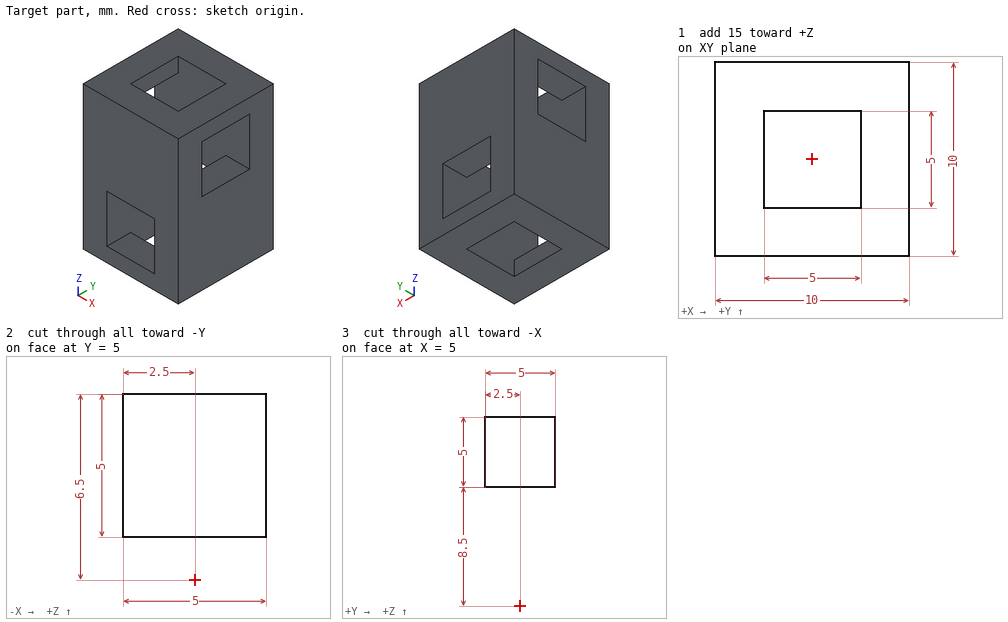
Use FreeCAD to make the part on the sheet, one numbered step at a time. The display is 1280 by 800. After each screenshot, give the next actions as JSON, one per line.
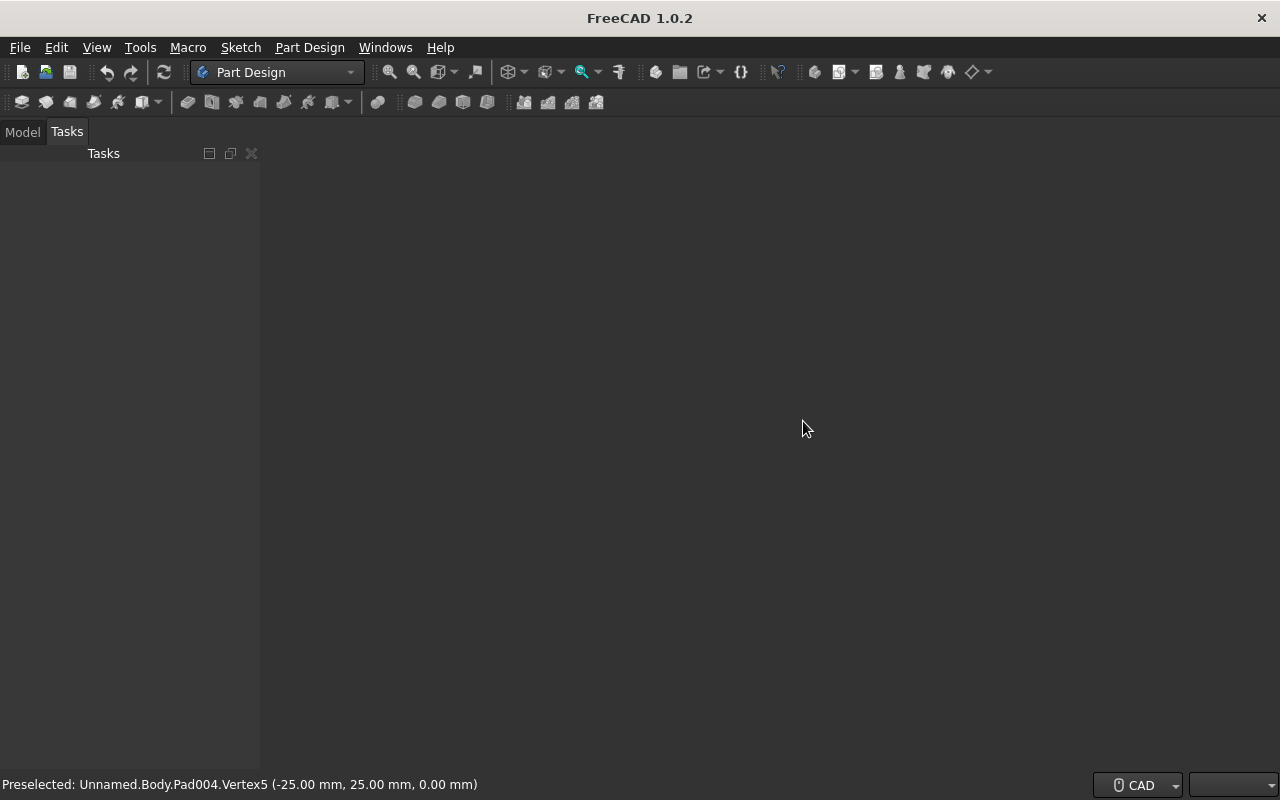
{"action": "left_click", "coordinate": [22, 72]}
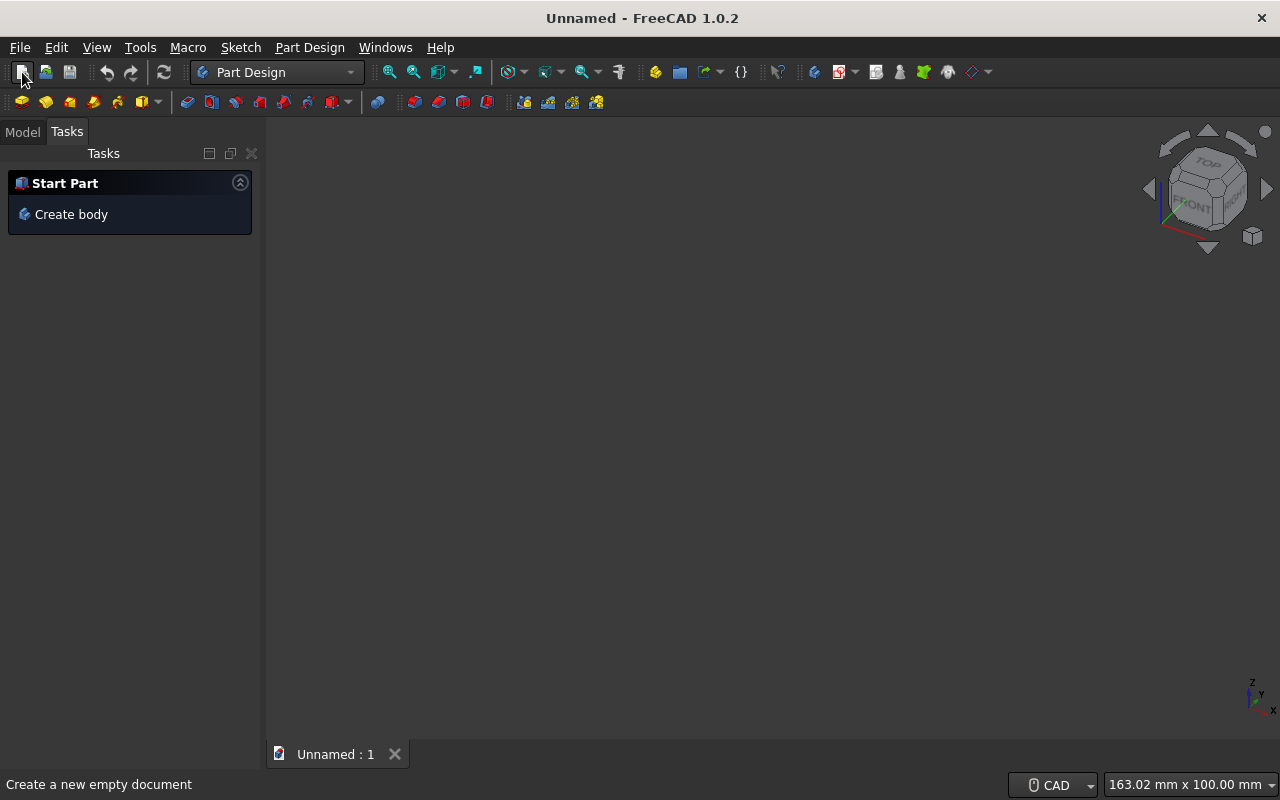
{"action": "left_click", "coordinate": [840, 72]}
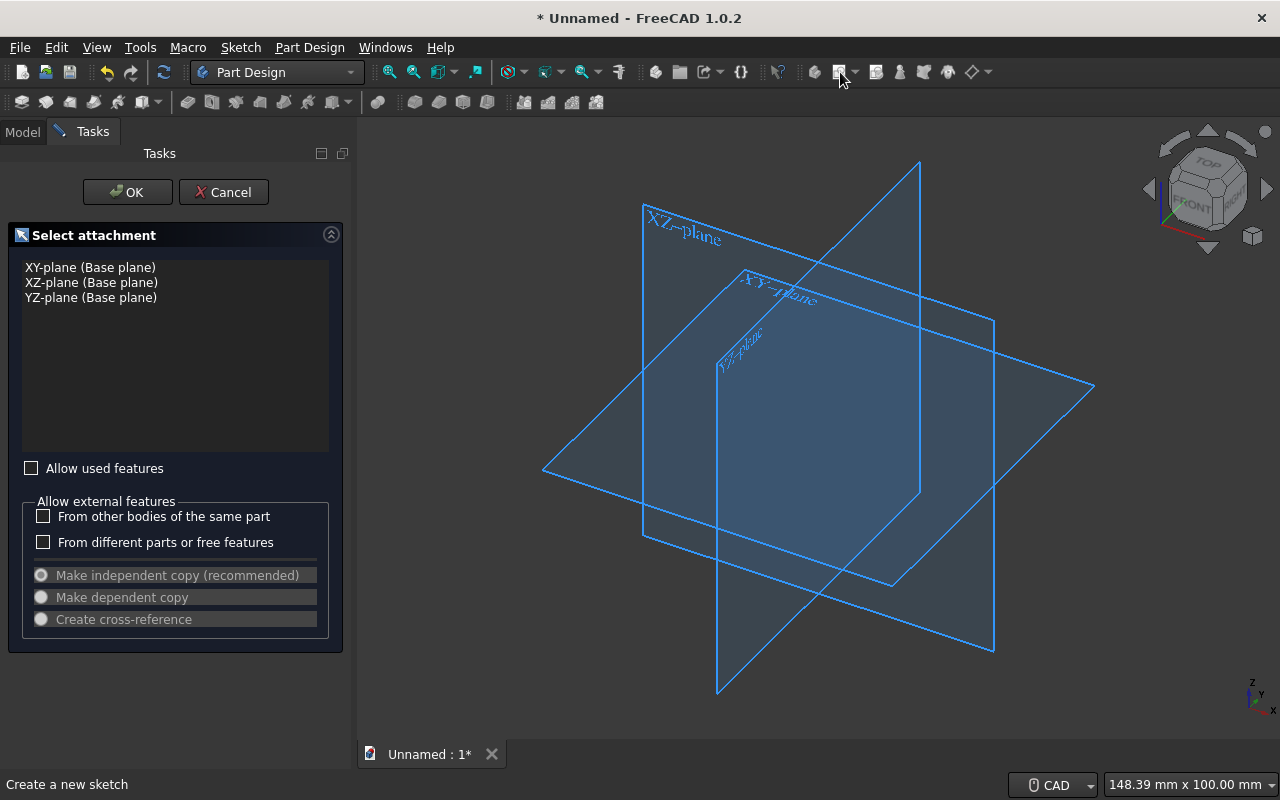
{"action": "left_click", "coordinate": [82, 268]}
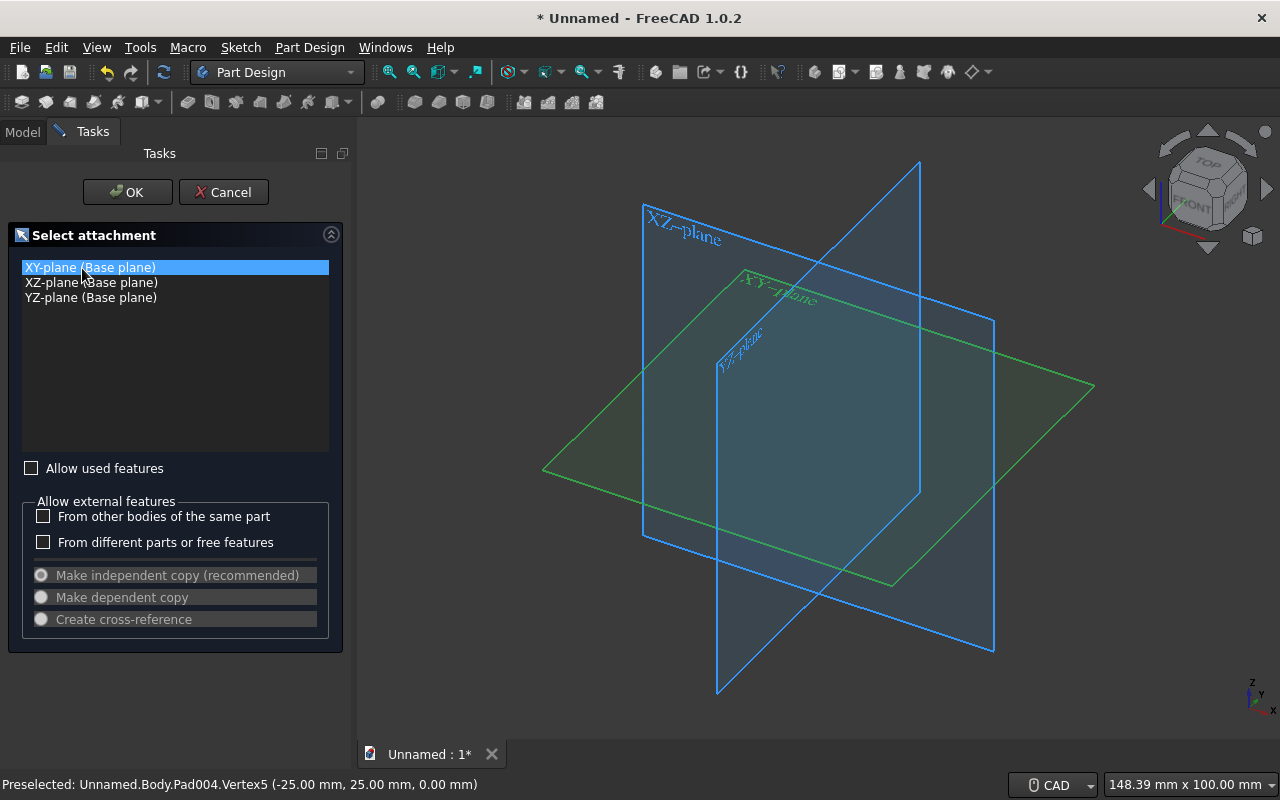
{"action": "left_click", "coordinate": [128, 192]}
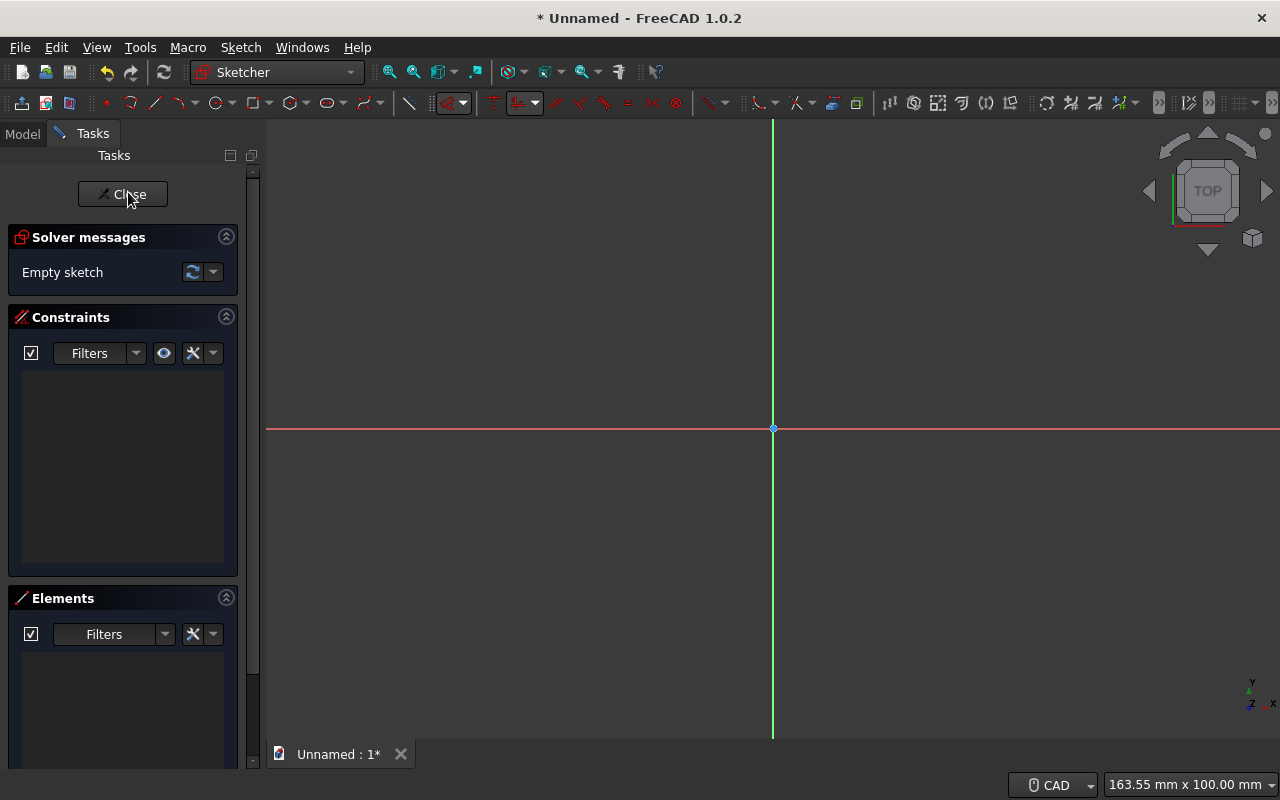
{"action": "scroll", "coordinate": [787, 429], "scroll_direction": "up", "scroll_amount": 9}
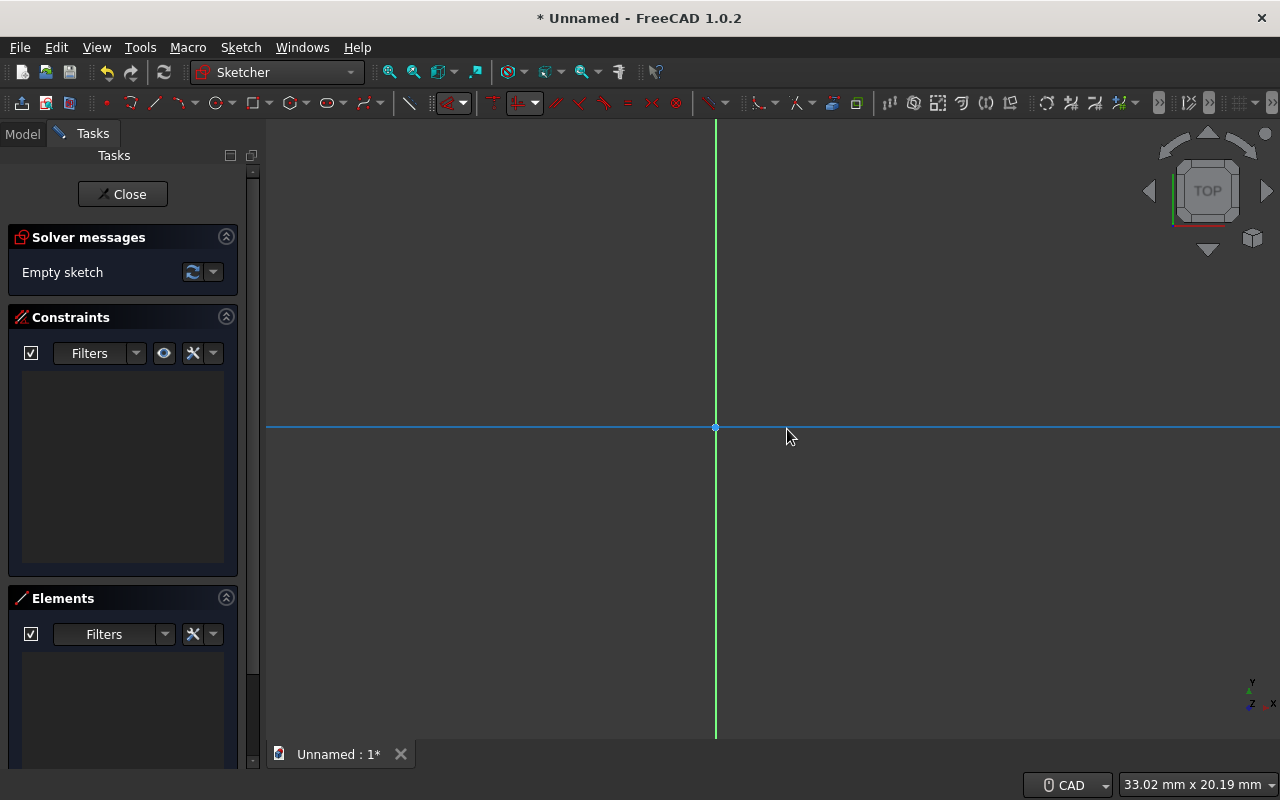
{"action": "left_click", "coordinate": [272, 104]}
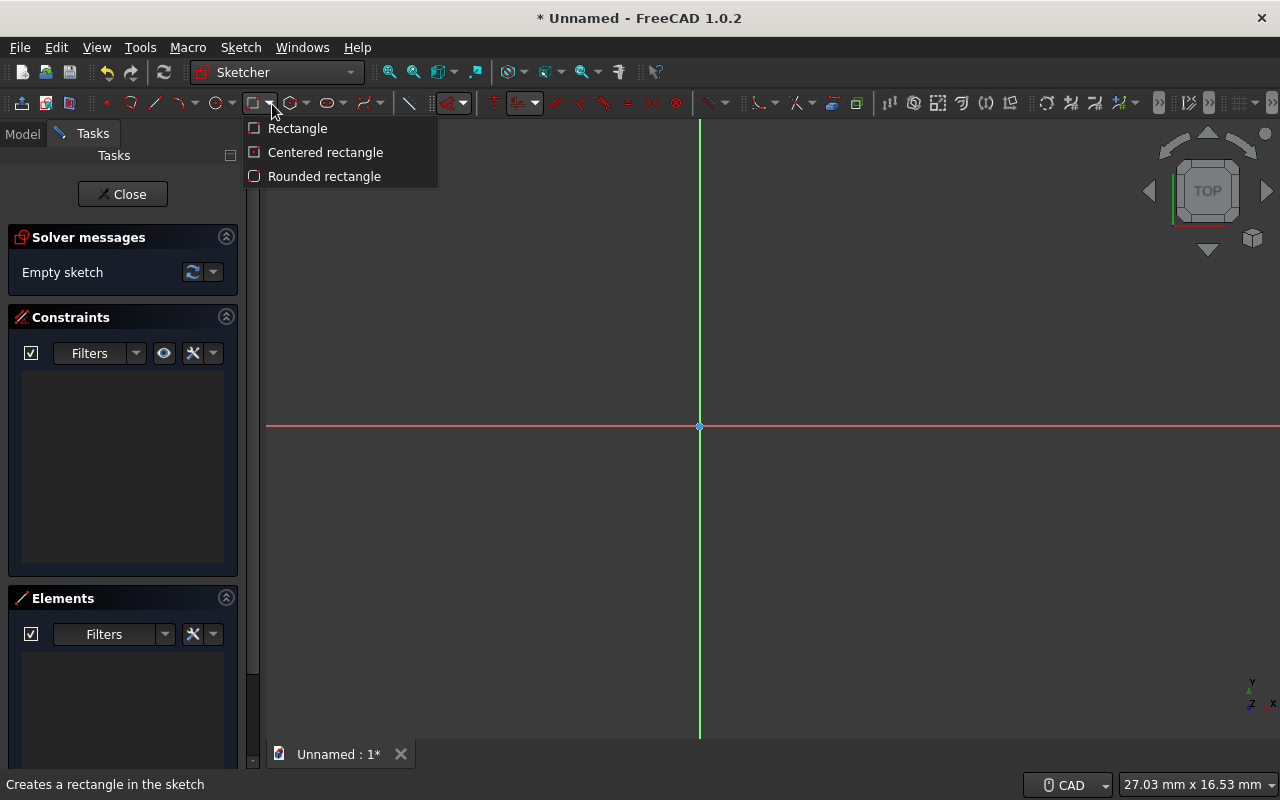
{"action": "left_click", "coordinate": [340, 152]}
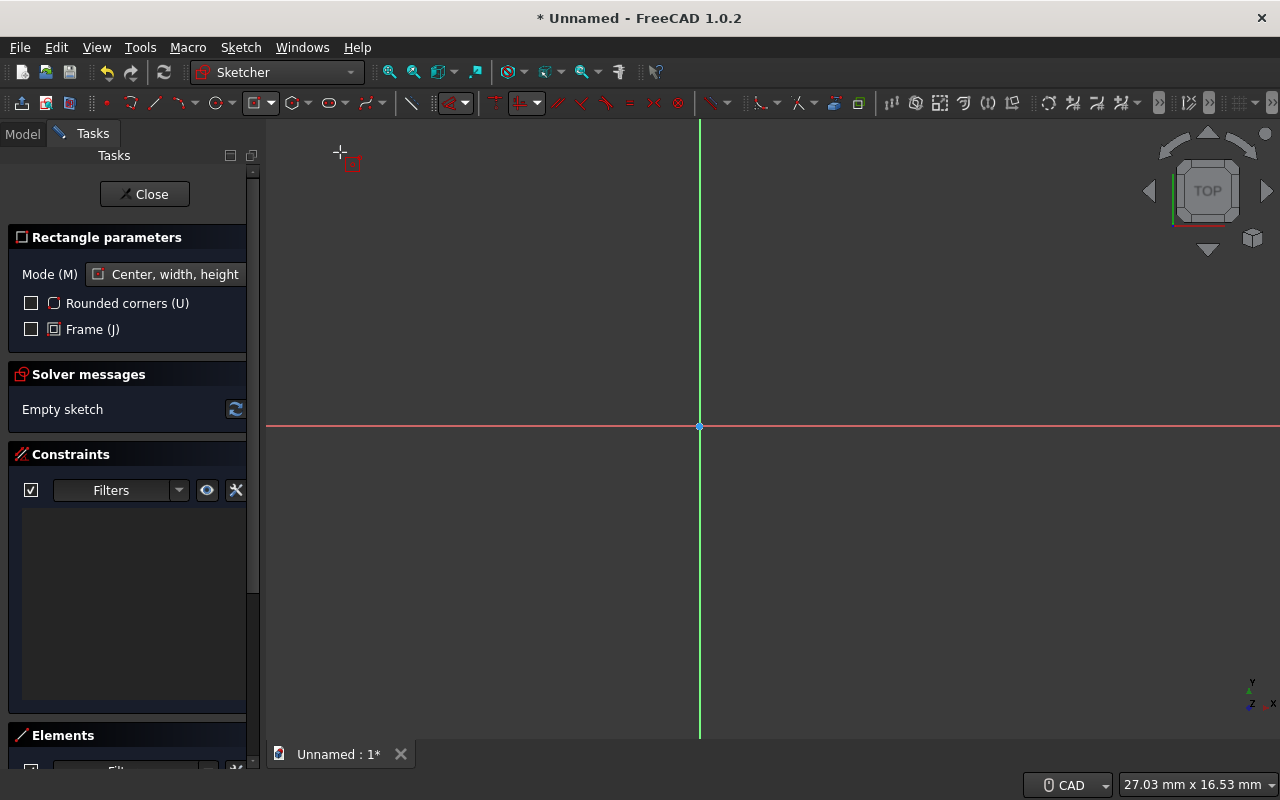
{"action": "left_click", "coordinate": [700, 426]}
{"action": "left_click", "coordinate": [887, 239]}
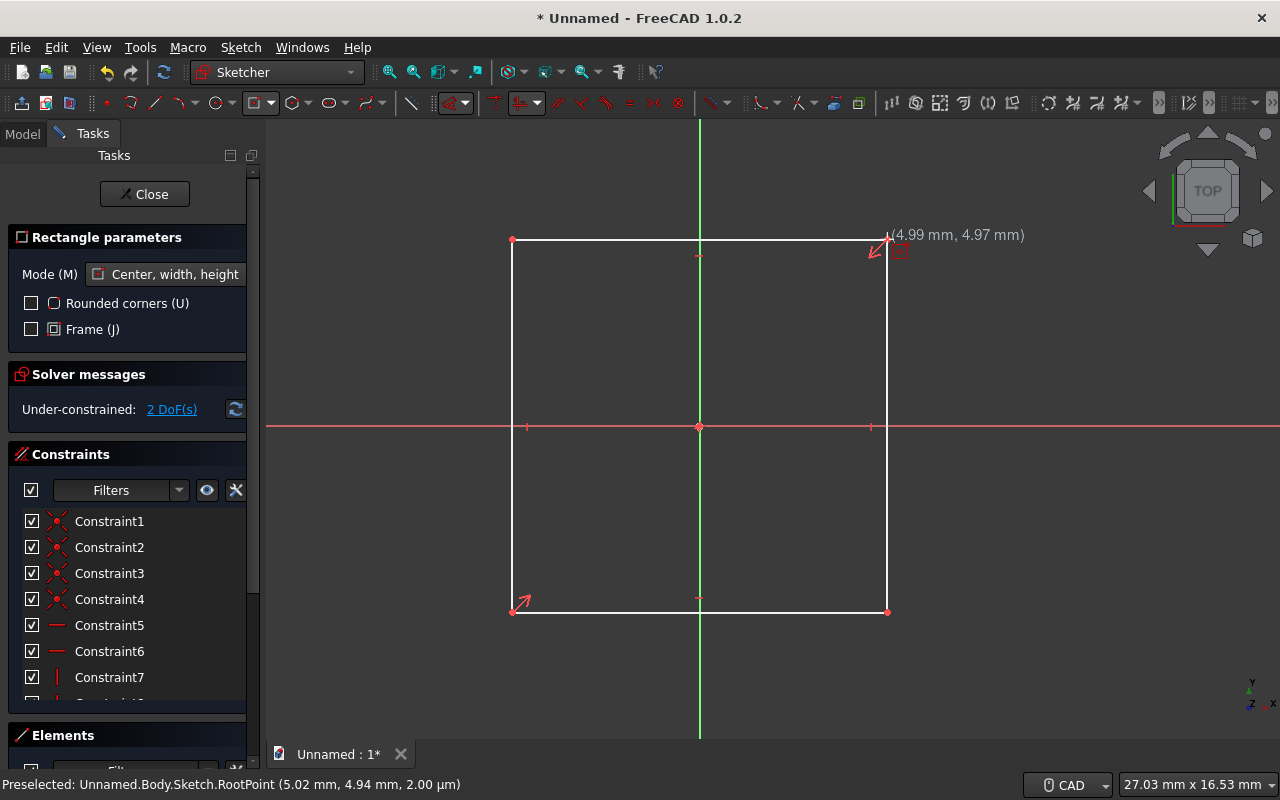
{"action": "left_click", "coordinate": [700, 426]}
{"action": "left_click", "coordinate": [793, 333]}
{"action": "key", "text": "Escape"}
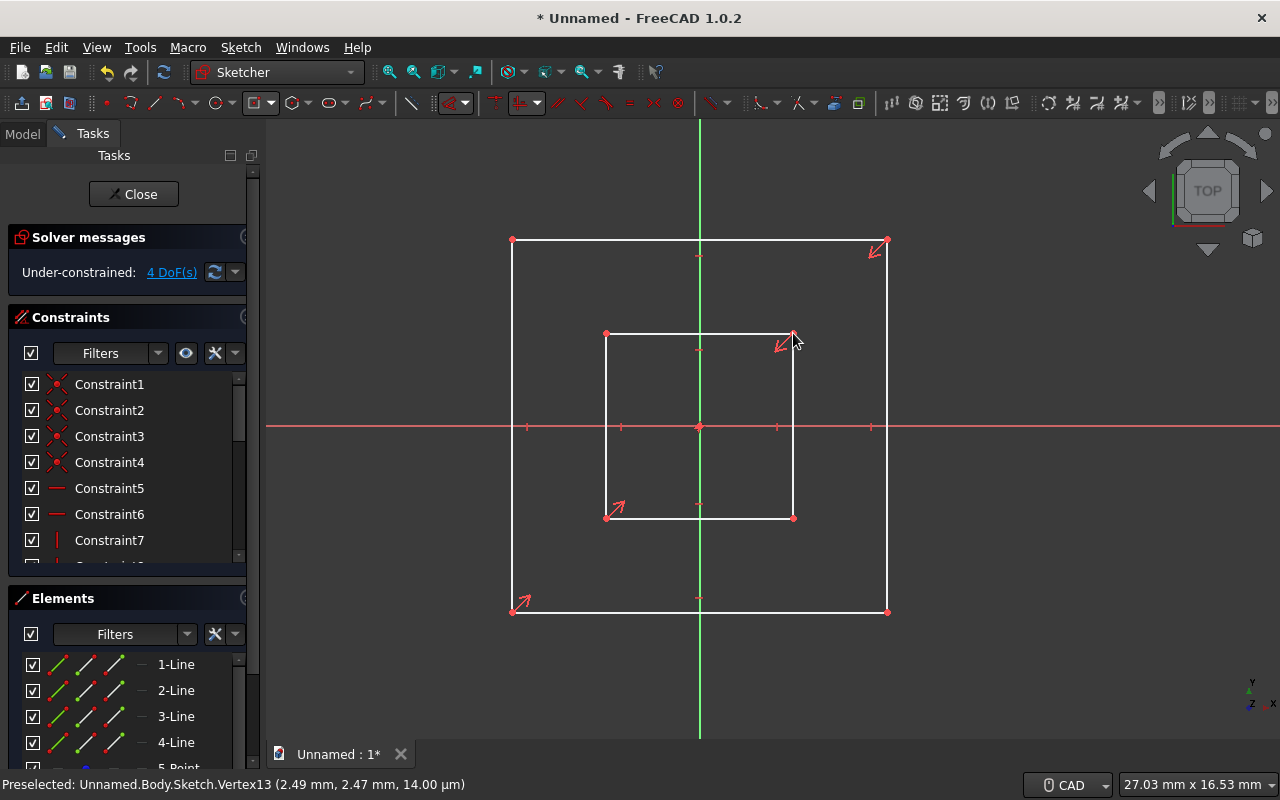
{"action": "left_click", "coordinate": [450, 104]}